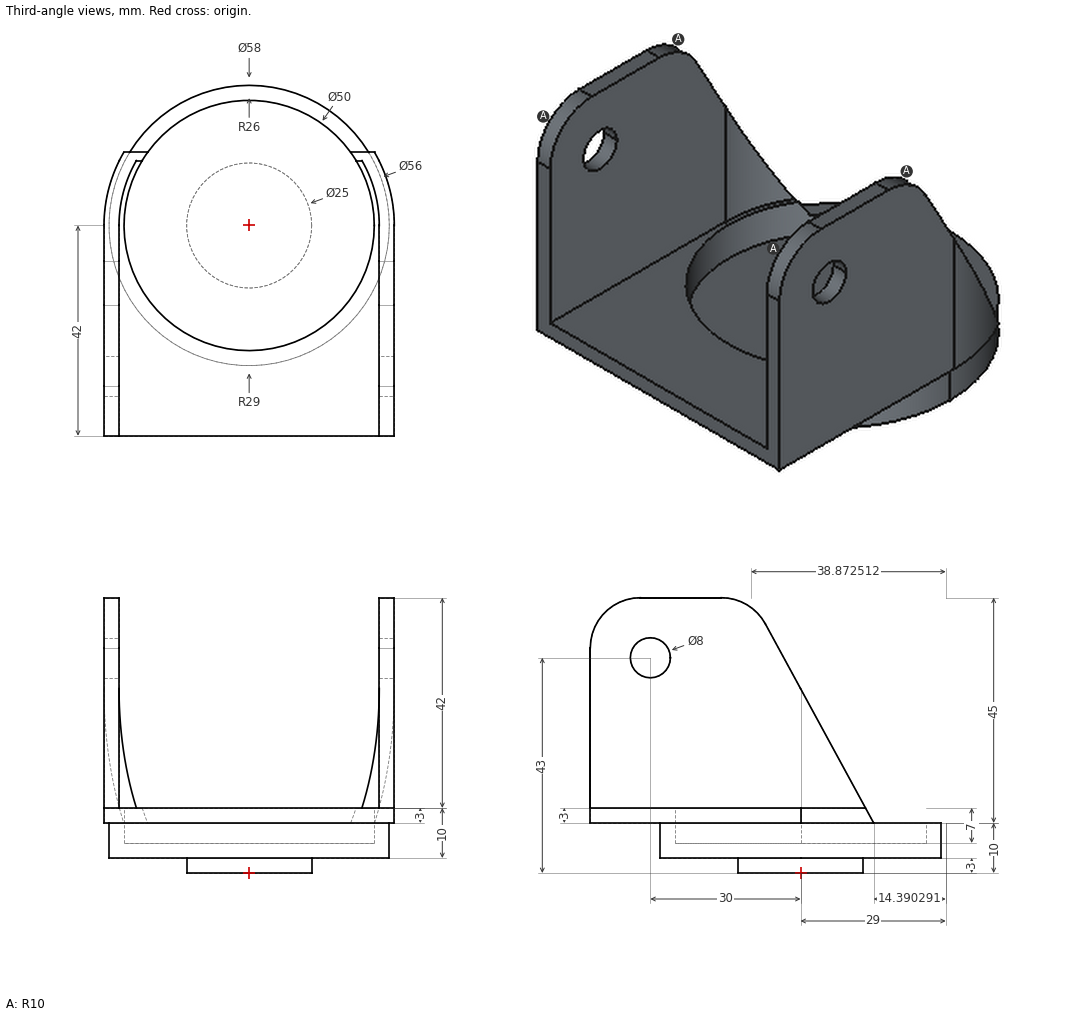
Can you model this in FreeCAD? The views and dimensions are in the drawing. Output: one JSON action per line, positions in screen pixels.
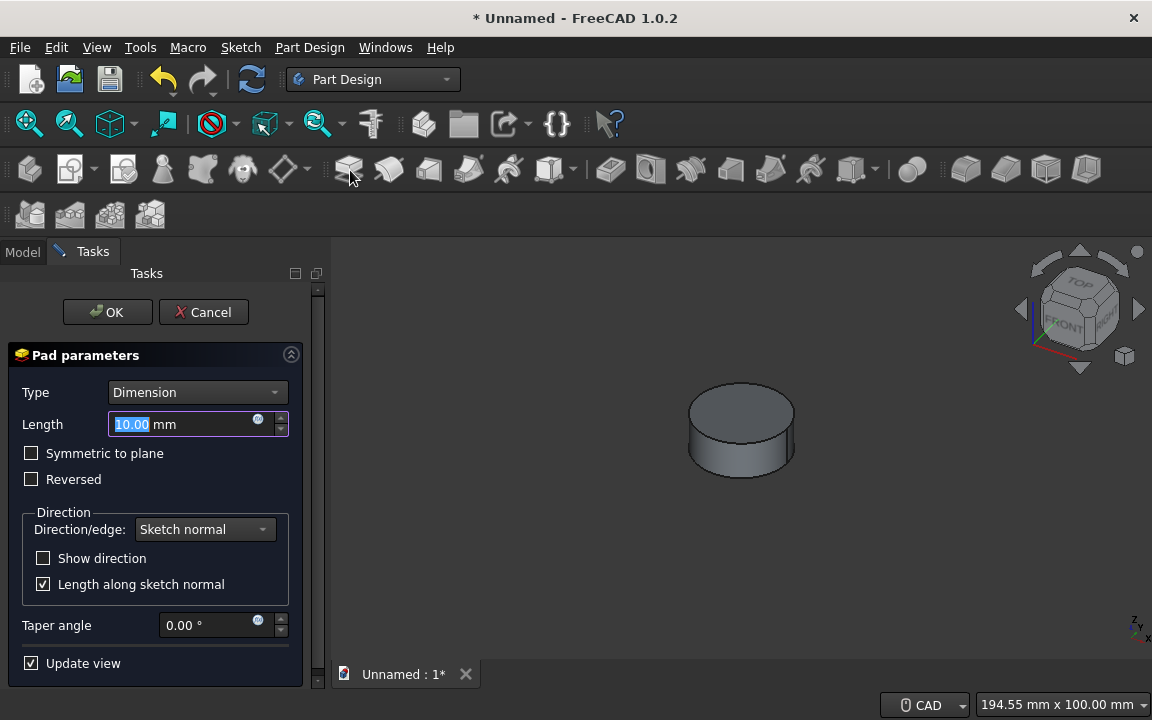
{"action": "type", "text": "3"}
{"action": "key", "text": "Tab"}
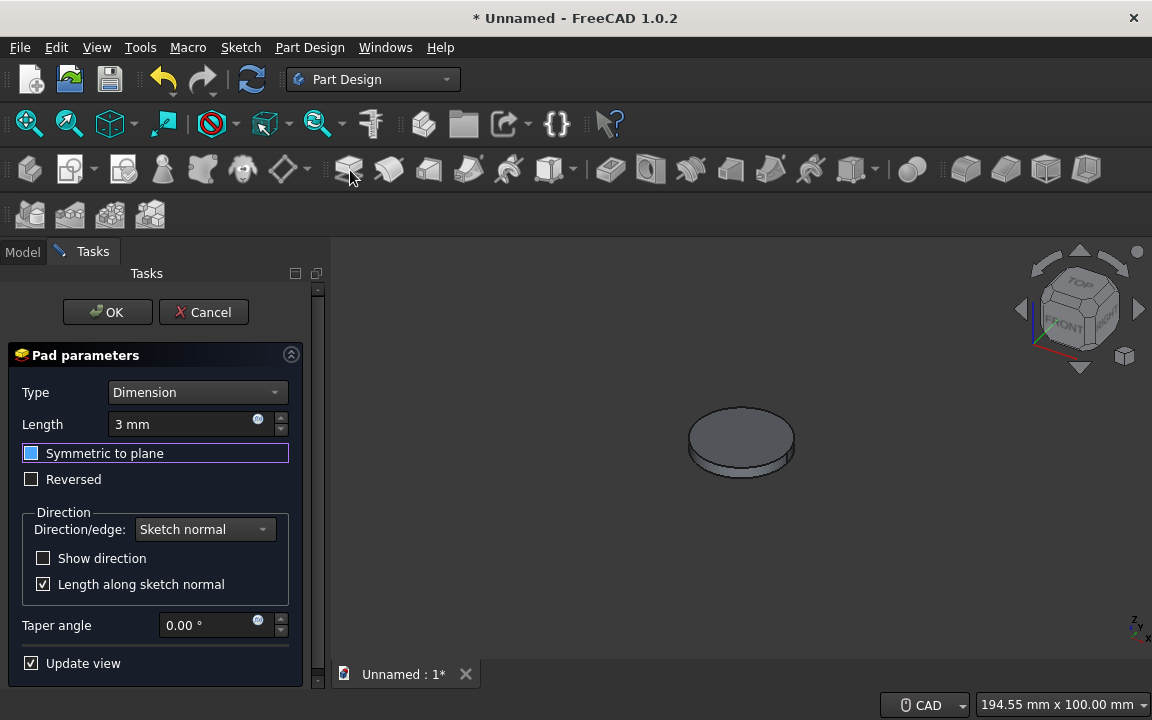
{"action": "left_click", "coordinate": [108, 312]}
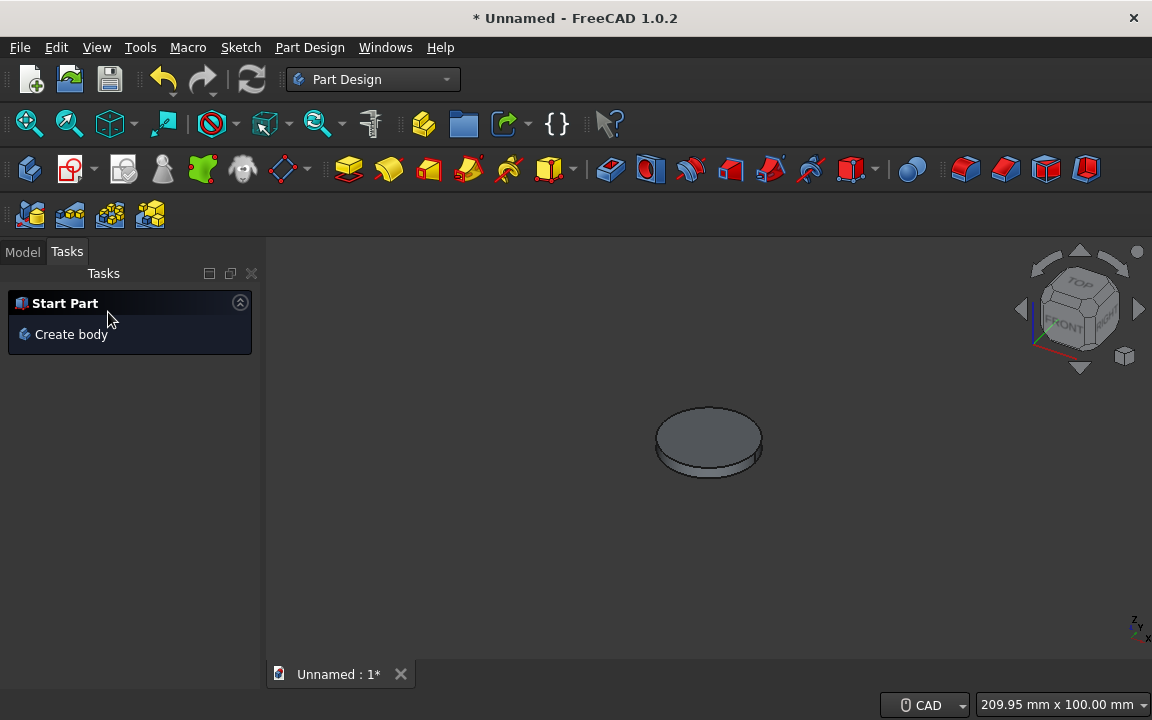
{"action": "left_click", "coordinate": [30, 124]}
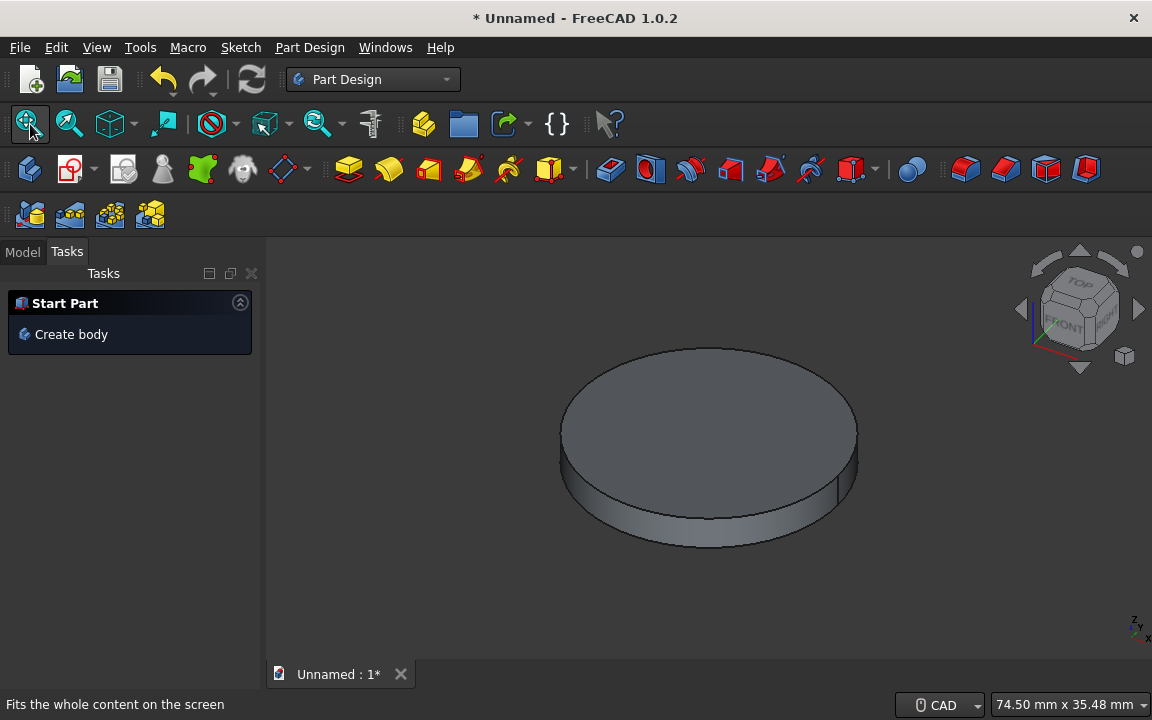
{"action": "left_click", "coordinate": [709, 432]}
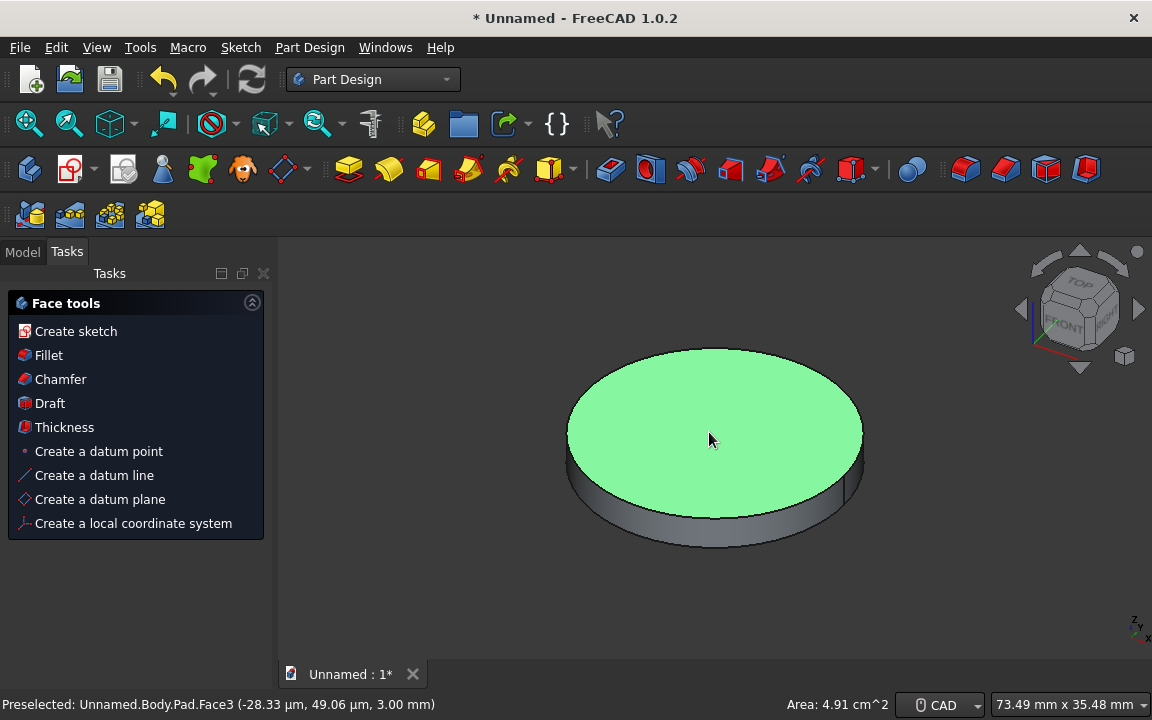
{"action": "left_click", "coordinate": [70, 170]}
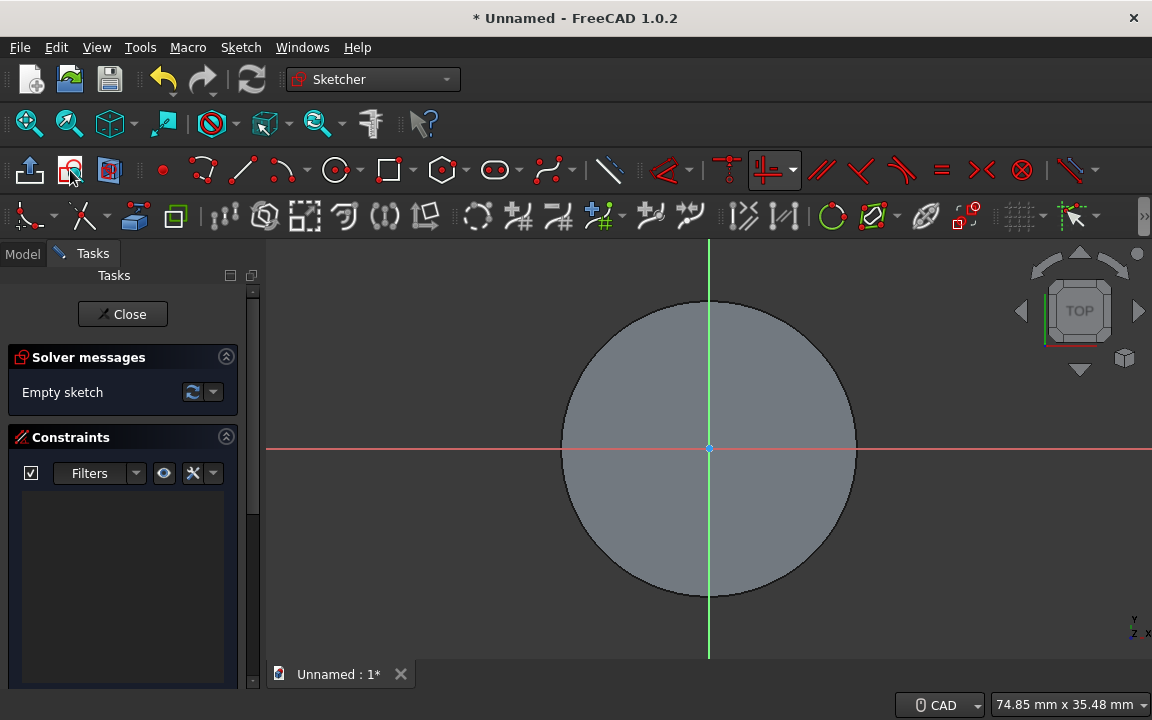
{"action": "scroll", "coordinate": [601, 449], "scroll_direction": "down", "scroll_amount": 5}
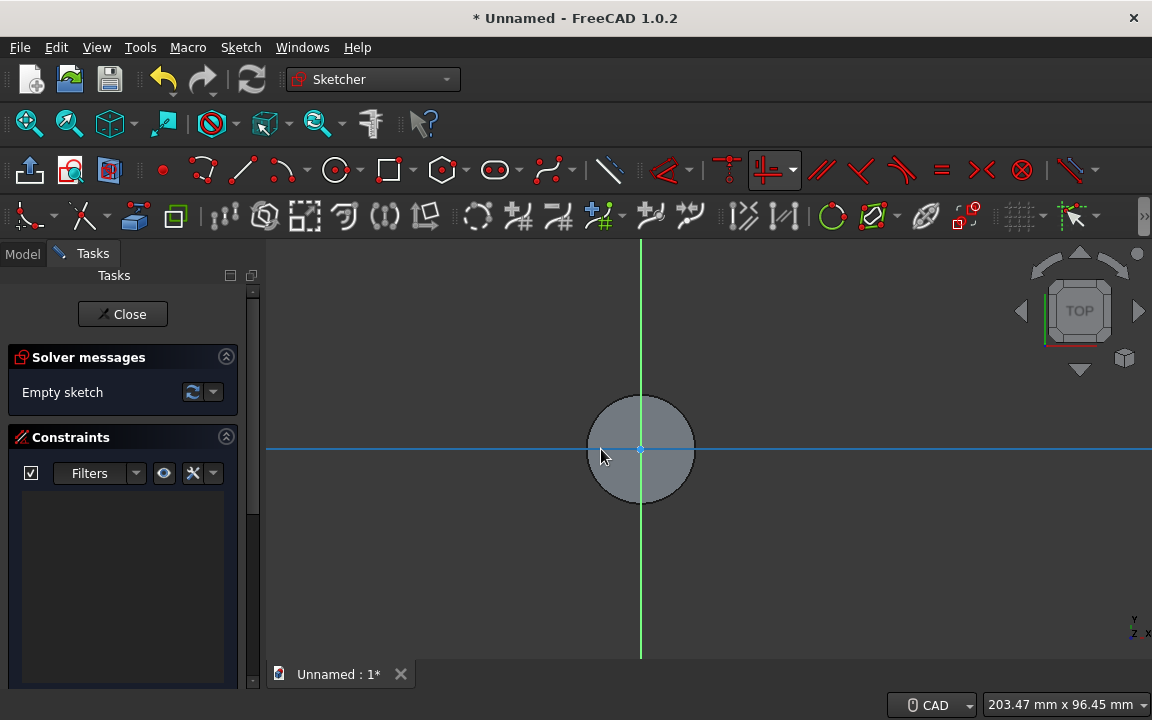
{"action": "left_click", "coordinate": [336, 170]}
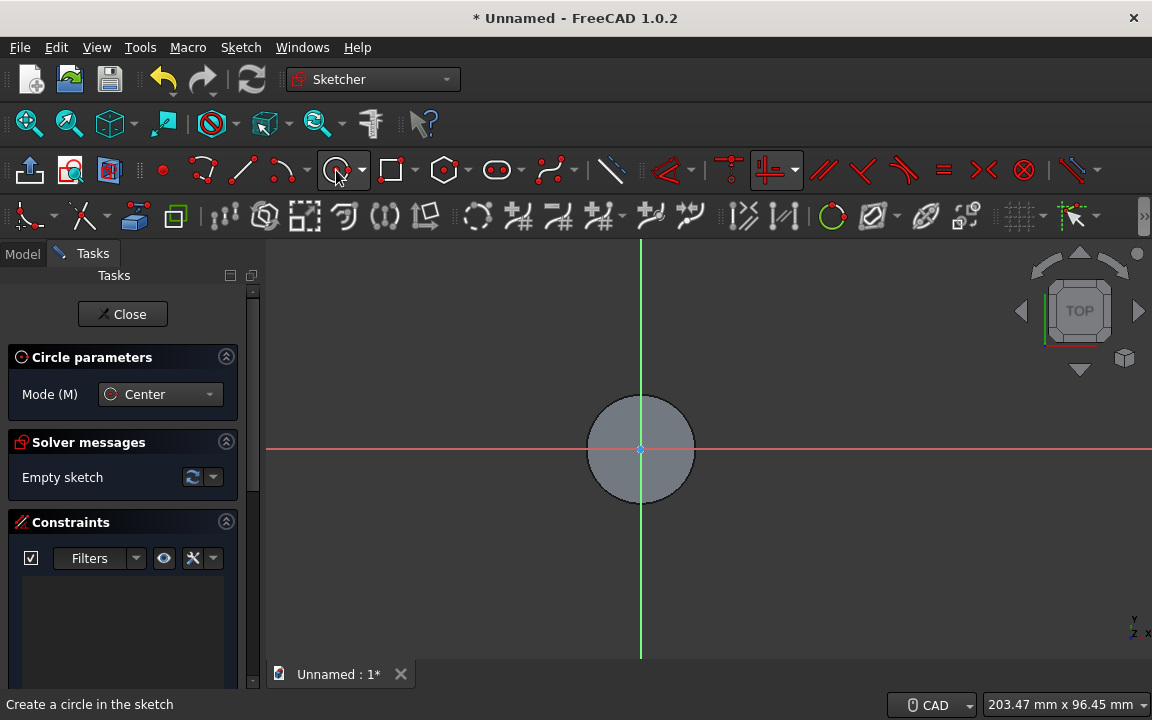
{"action": "left_click", "coordinate": [641, 449]}
{"action": "left_click", "coordinate": [727, 363]}
{"action": "key", "text": "Escape"}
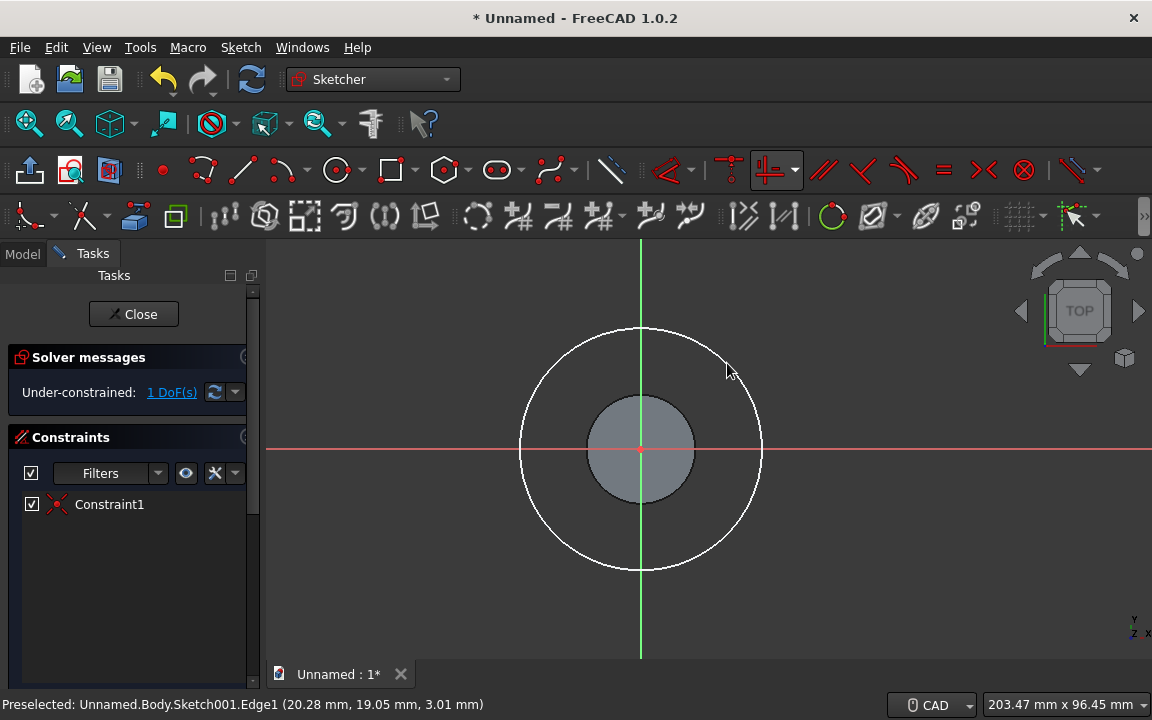
{"action": "left_click", "coordinate": [666, 170]}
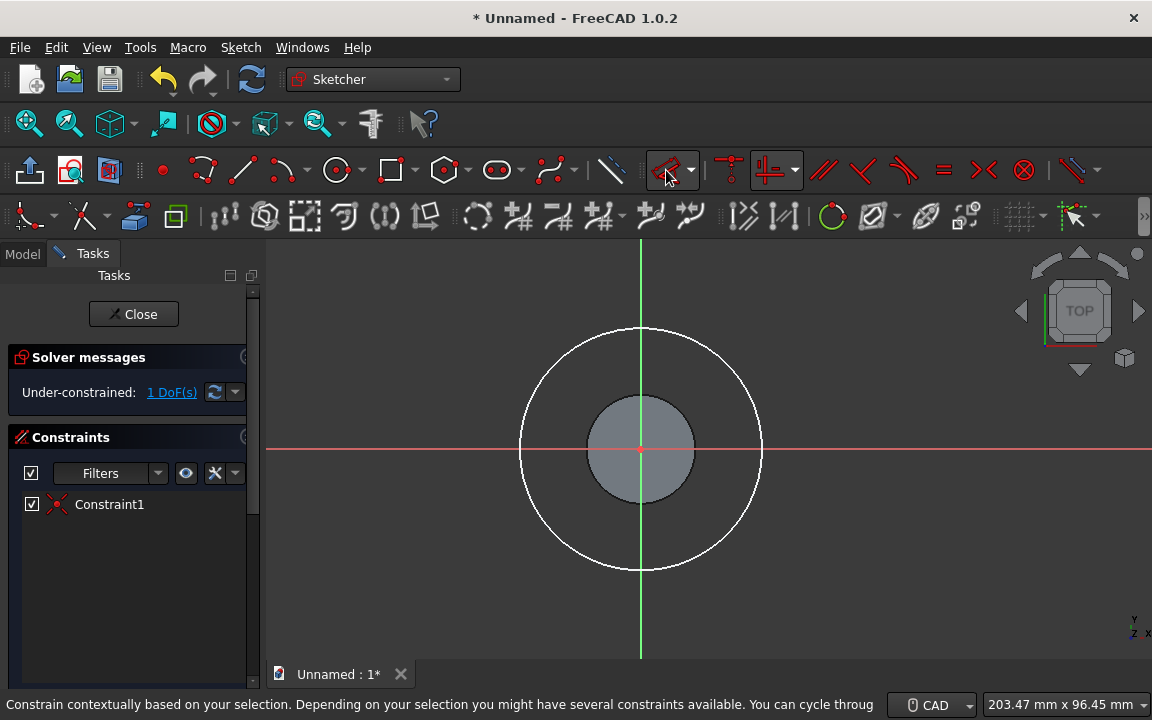
{"action": "left_click", "coordinate": [726, 363]}
{"action": "left_click", "coordinate": [748, 340]}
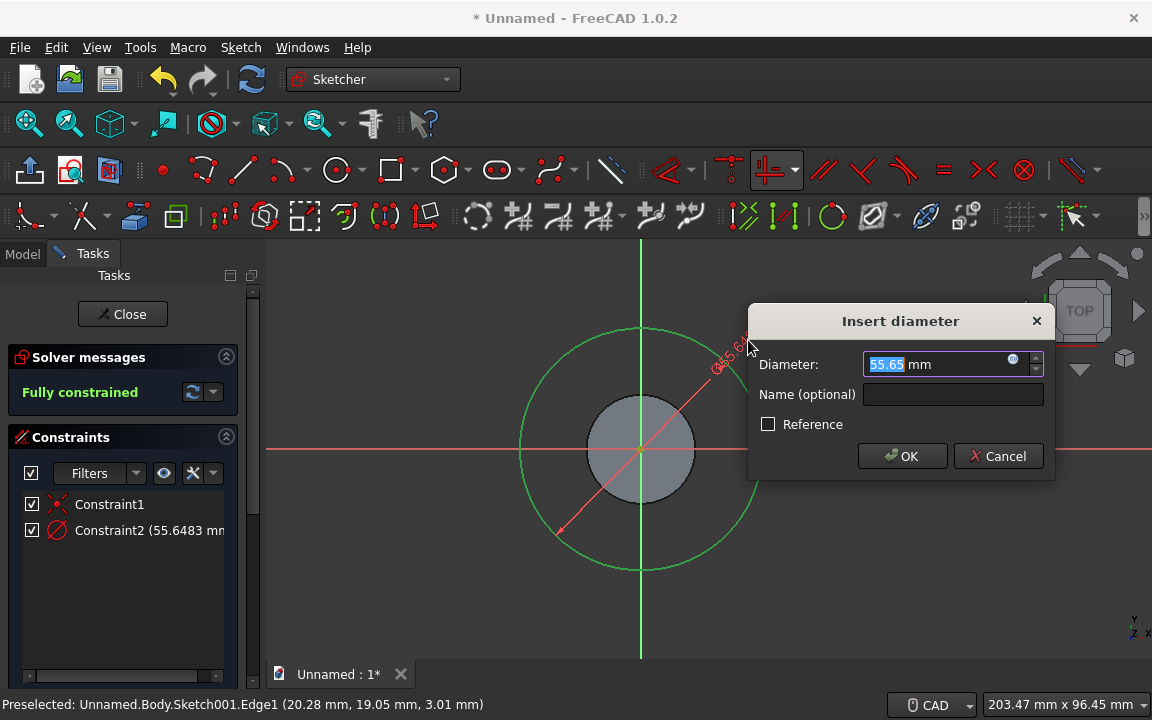
{"action": "type", "text": "56"}
{"action": "key", "text": "Return"}
{"action": "key", "text": "Escape"}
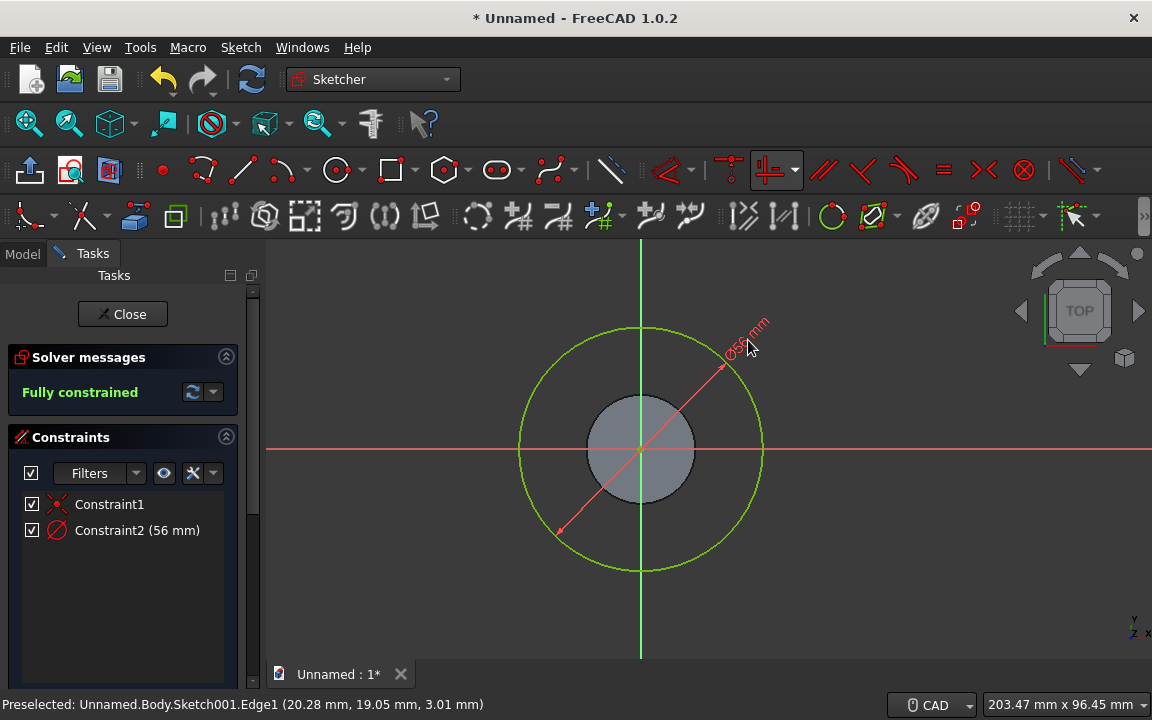
{"action": "left_click", "coordinate": [123, 314]}